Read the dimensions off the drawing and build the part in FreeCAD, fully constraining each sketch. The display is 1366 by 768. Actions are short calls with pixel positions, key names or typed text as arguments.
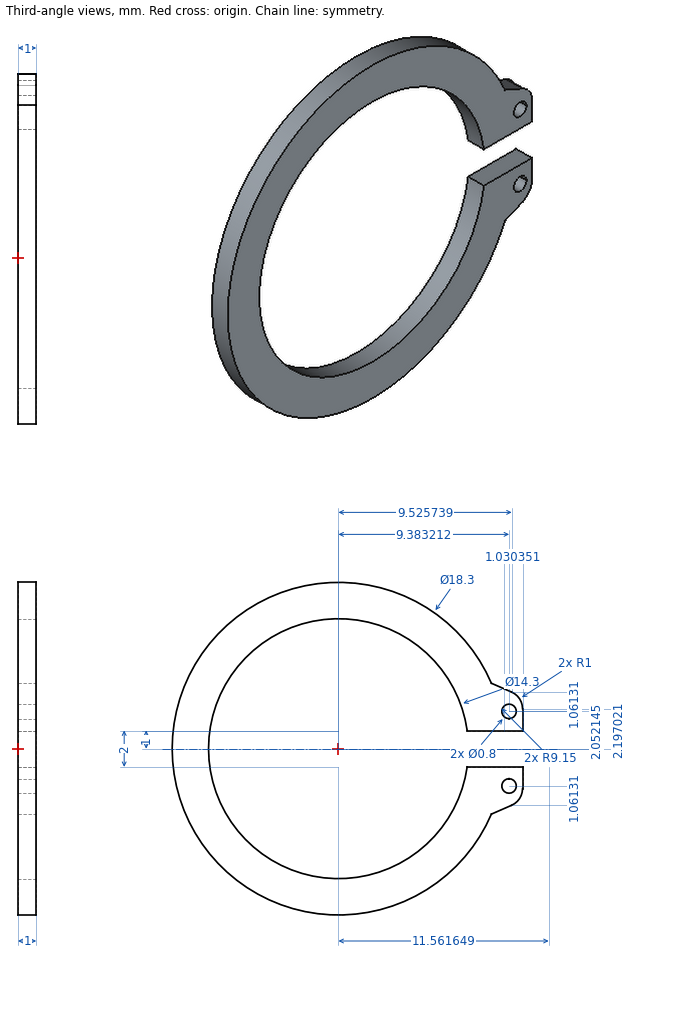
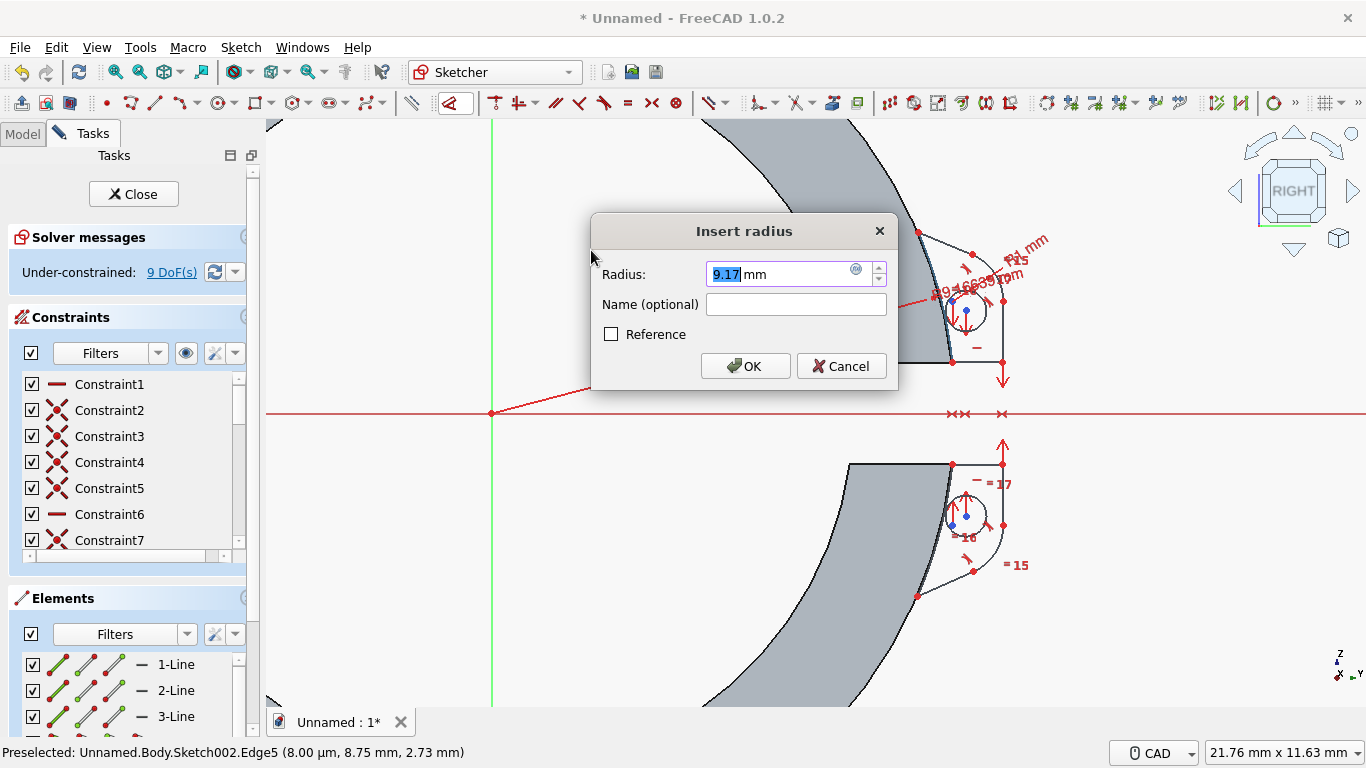
text(9.15)
key(Return)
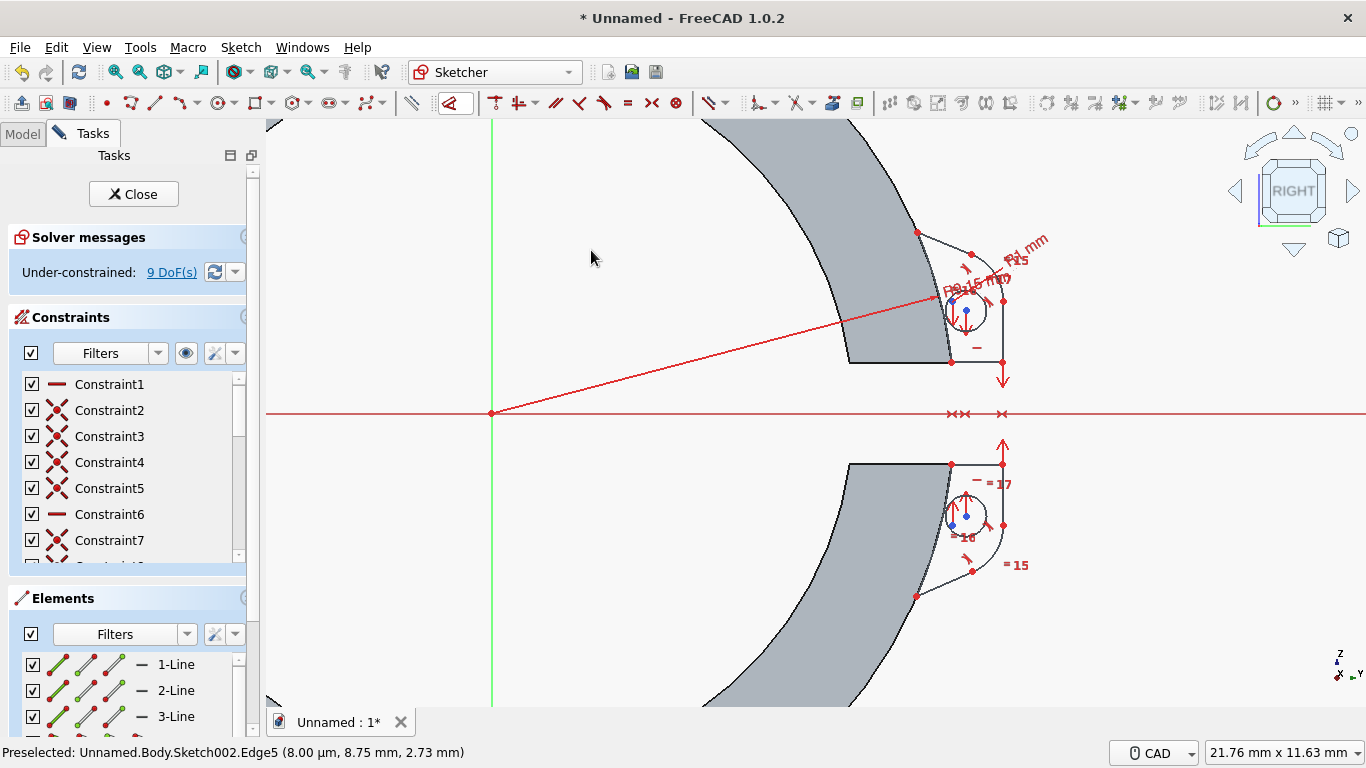
click(980, 296)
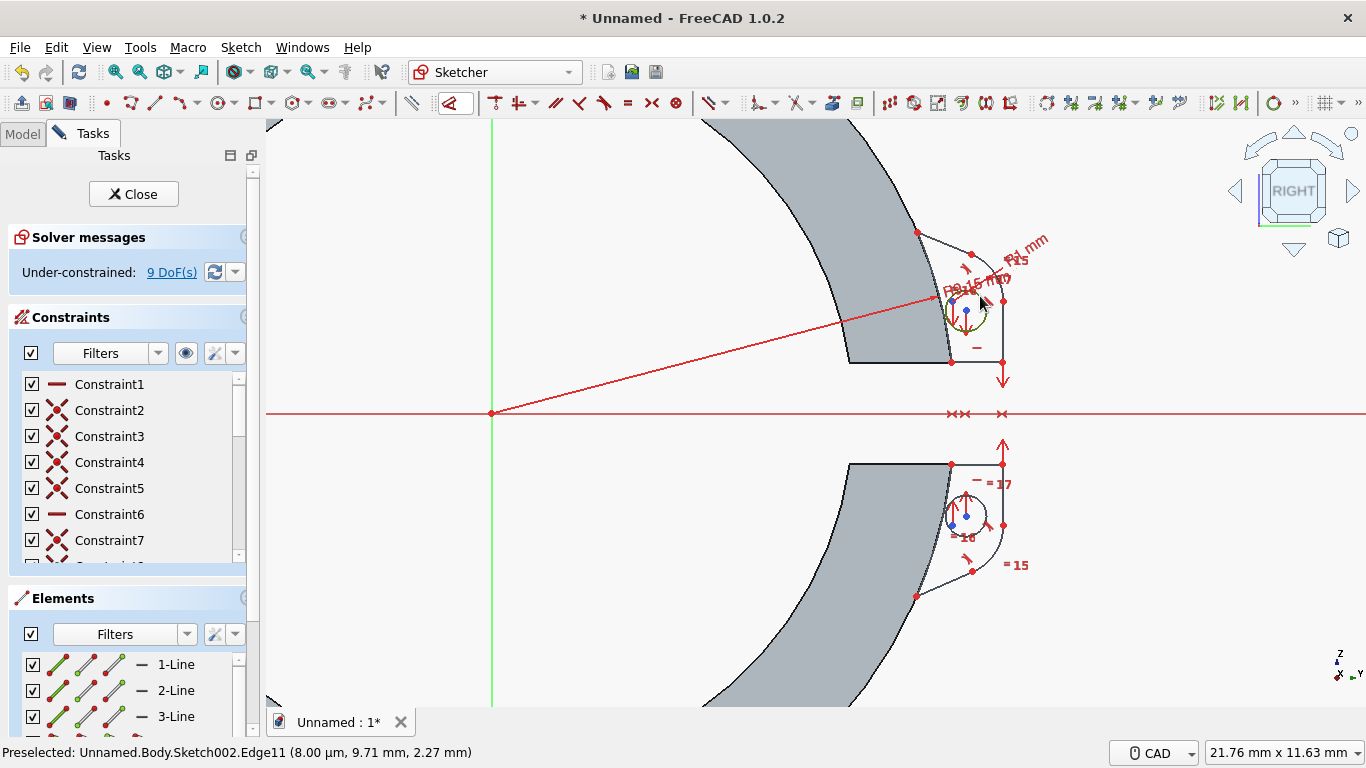
key(k)
key(o)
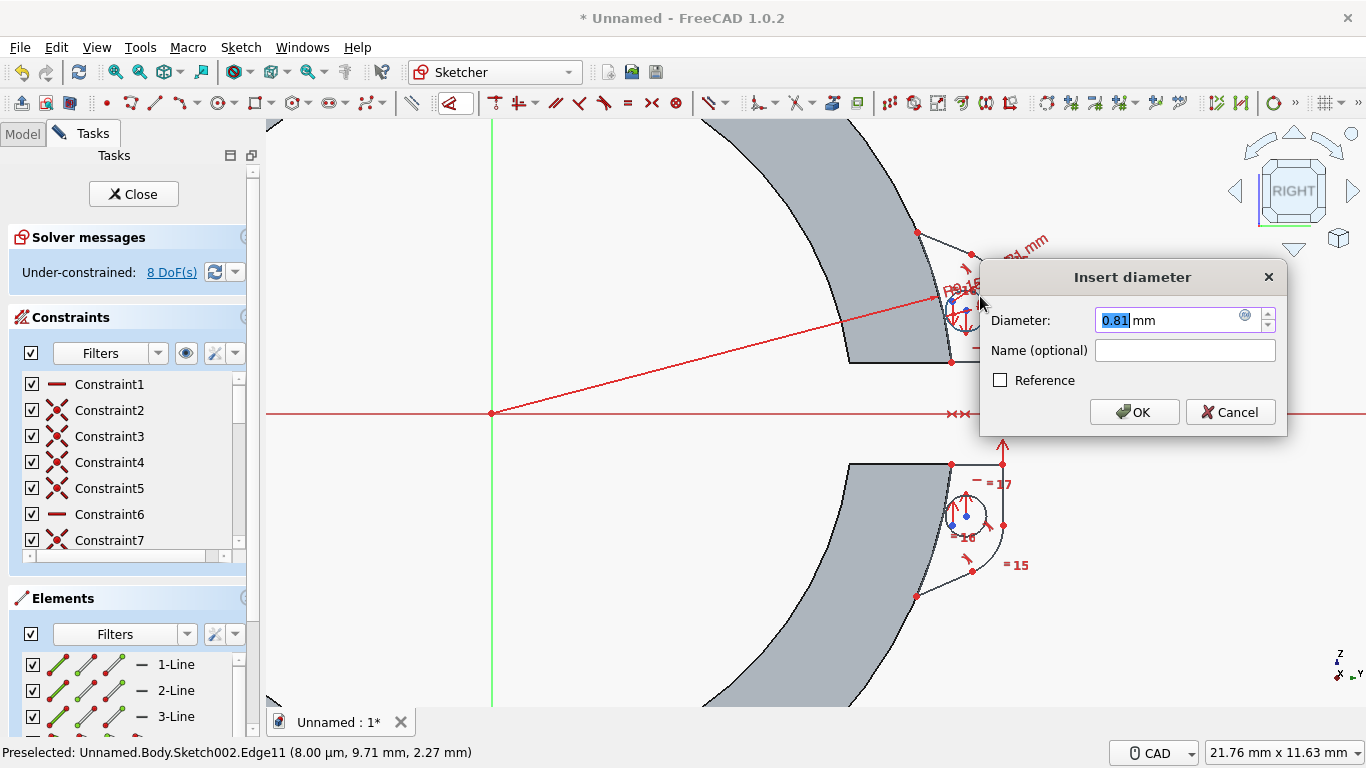
text(0.8)
key(Return)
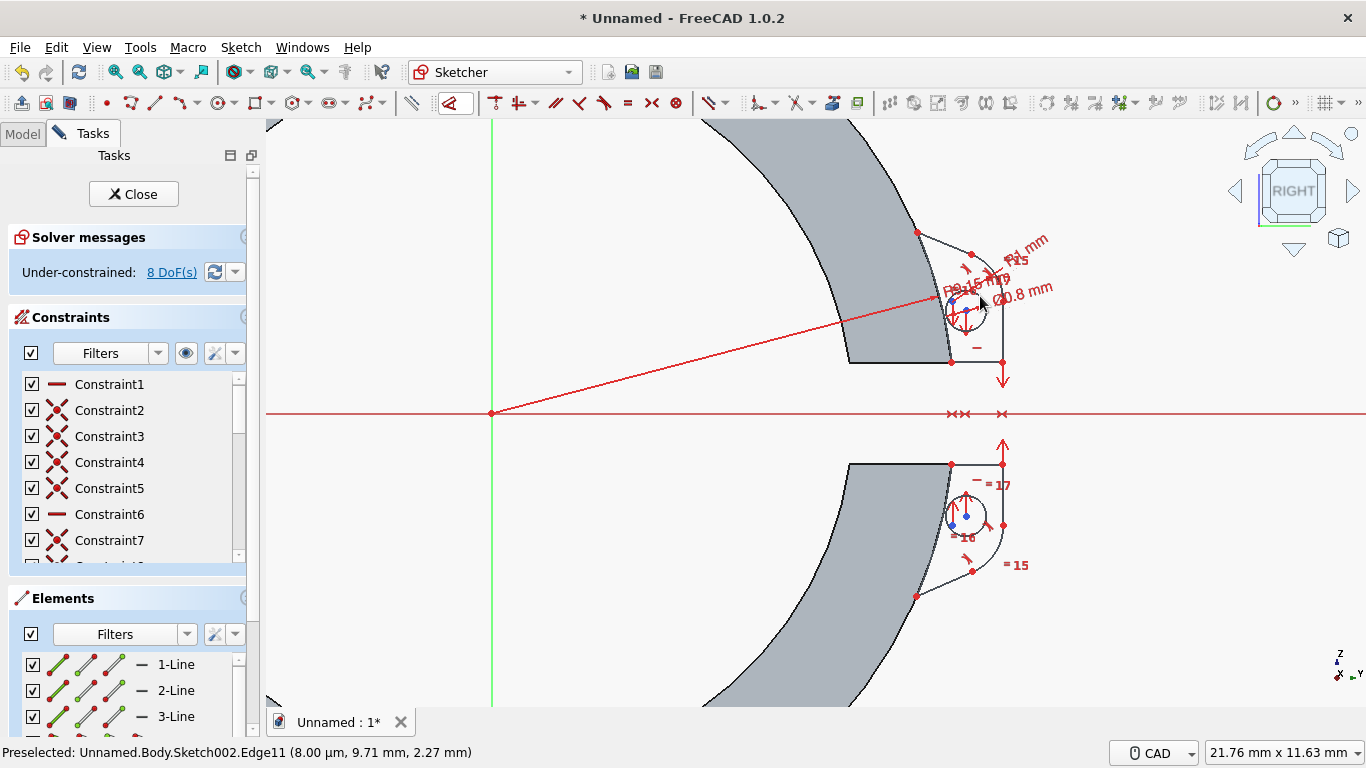
click(952, 362)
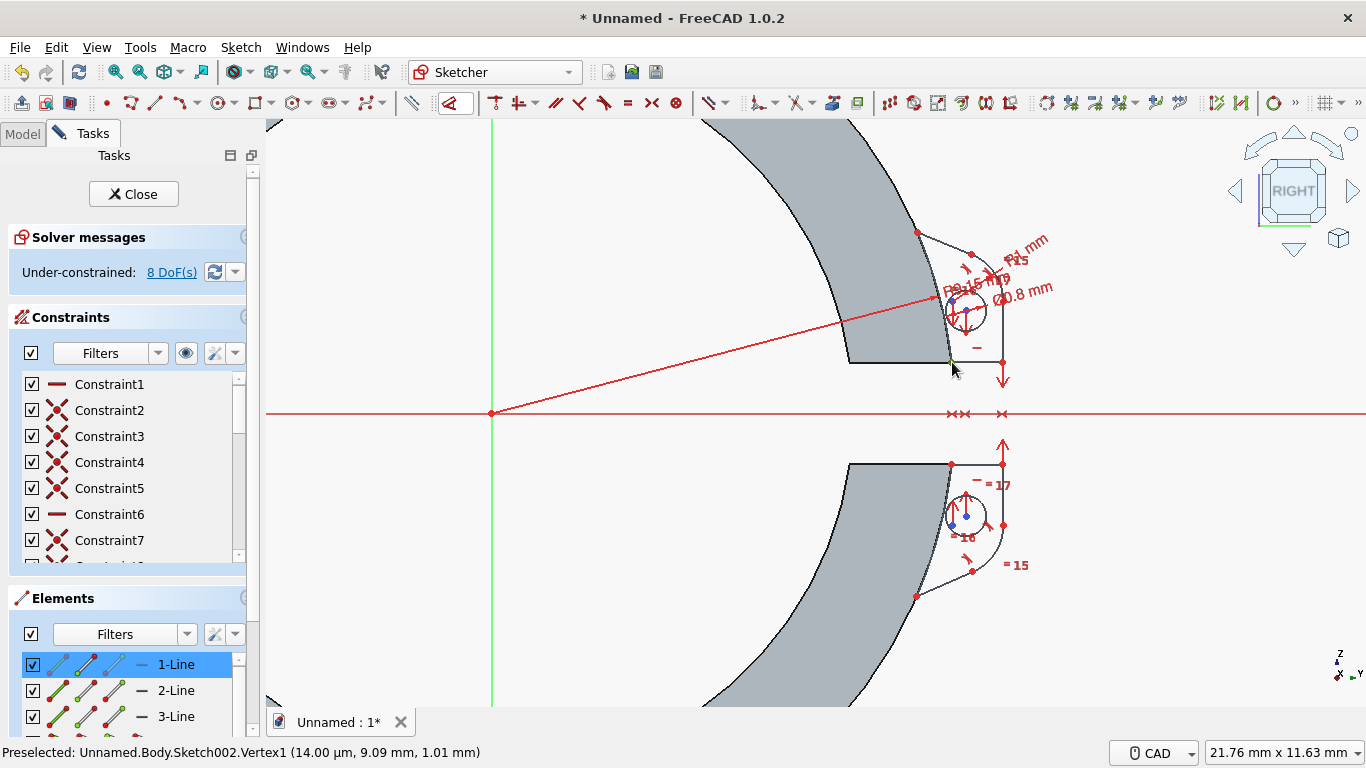
key(i)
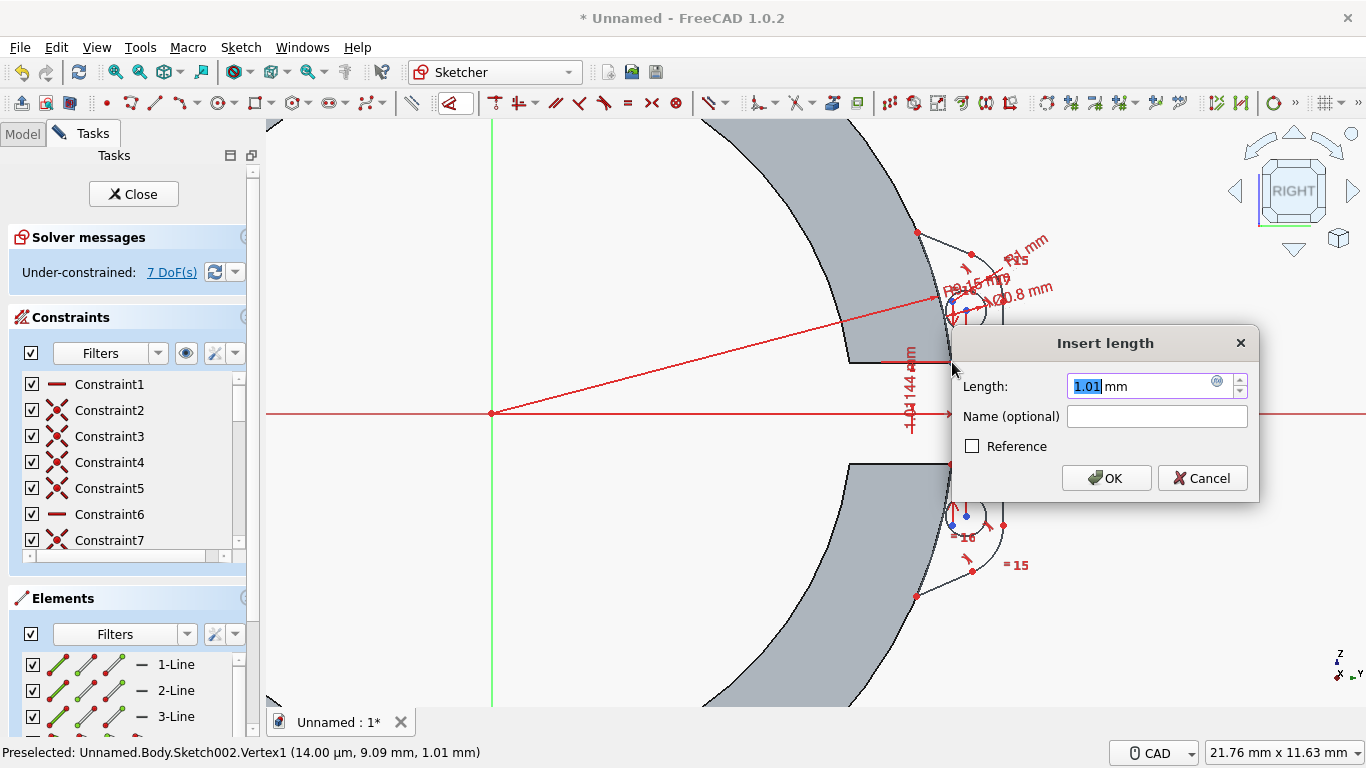
text(1)
key(Return)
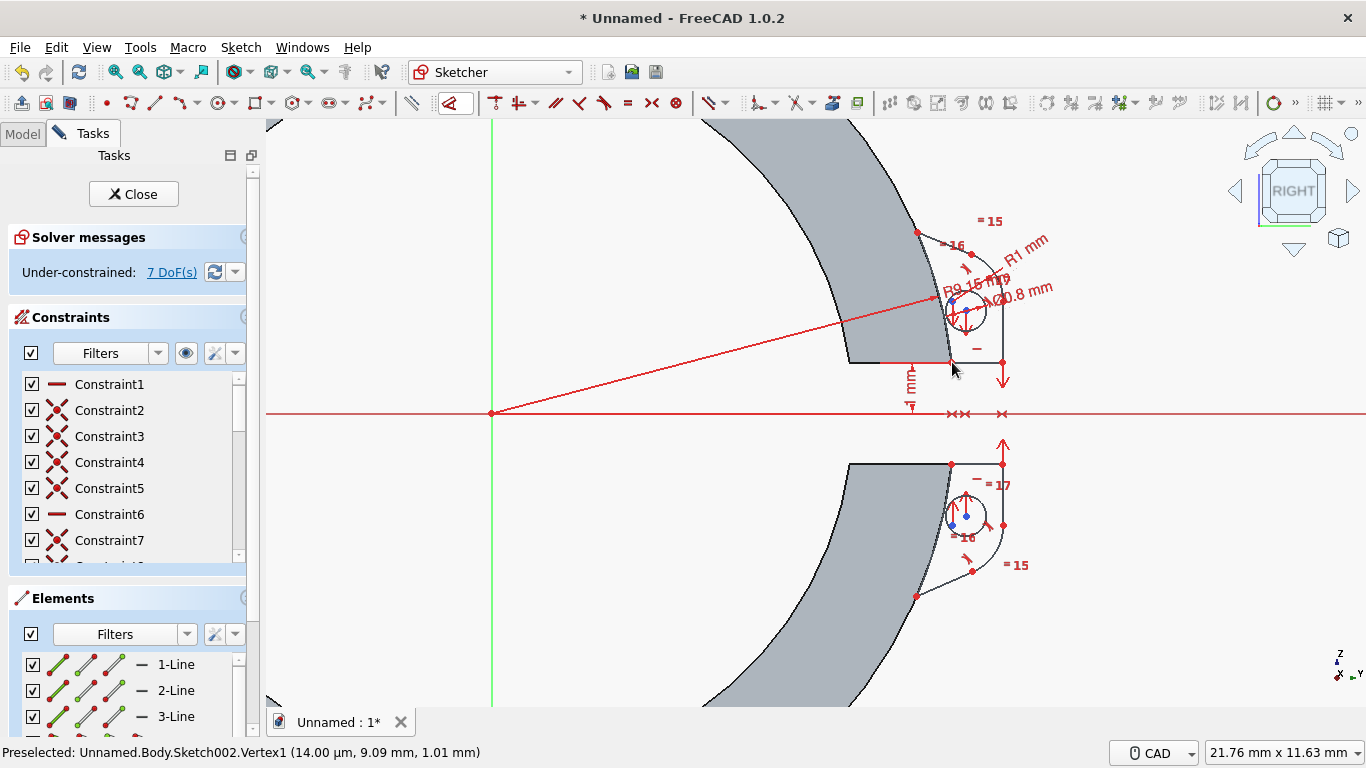
click(967, 363)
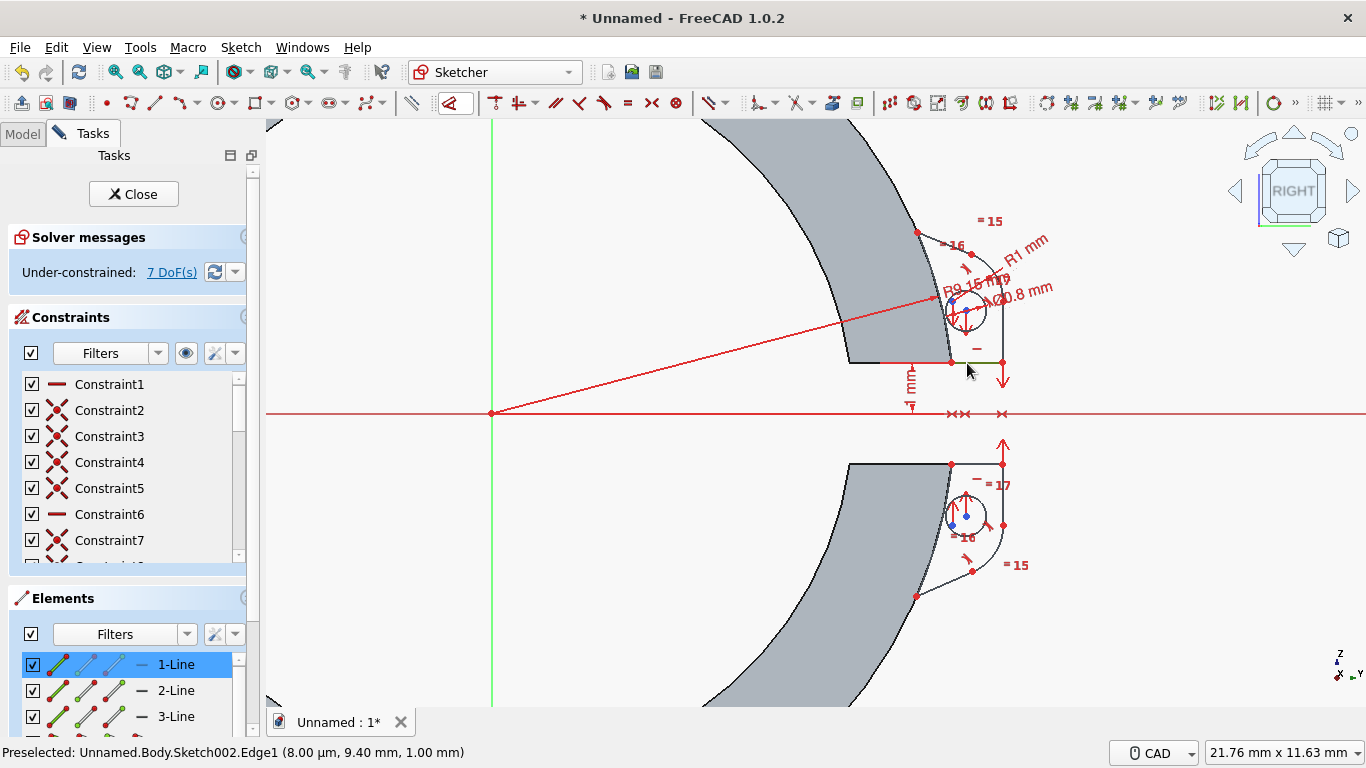
key(l)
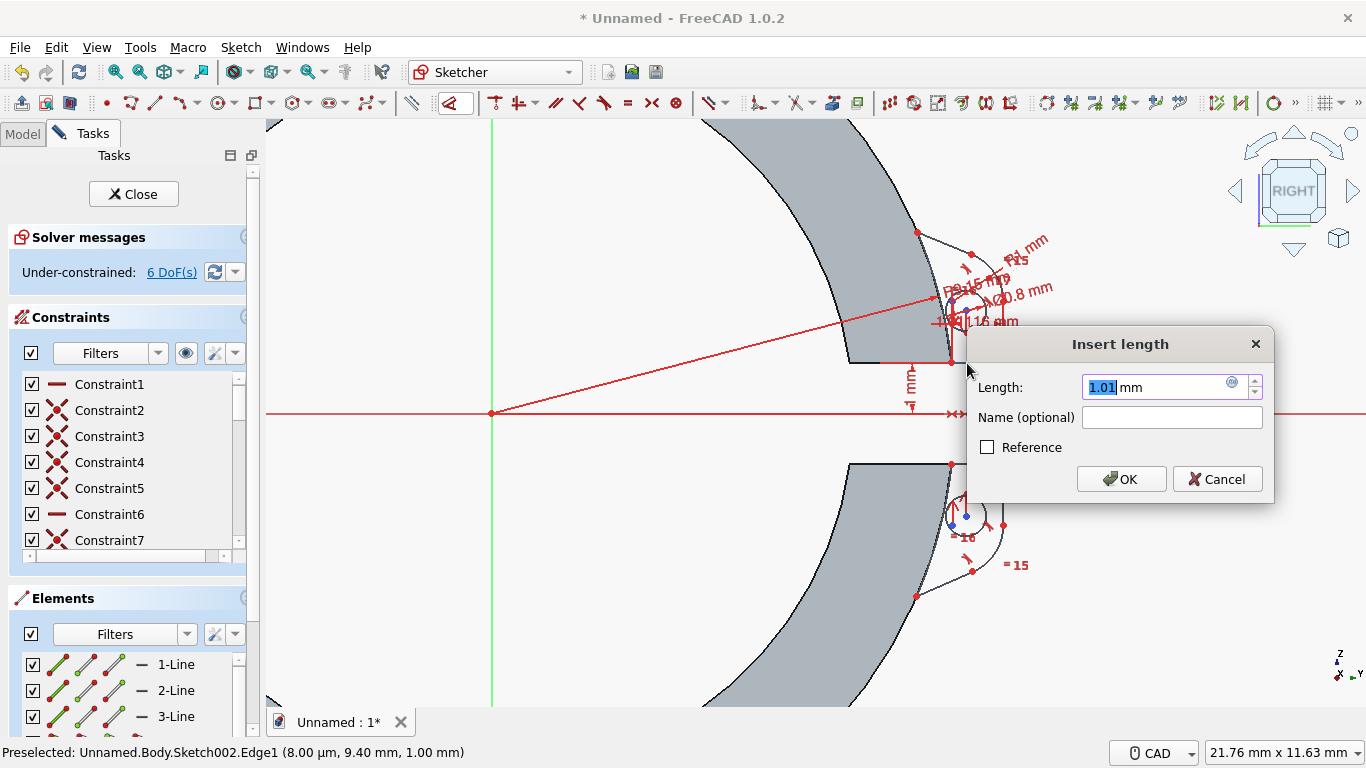
text(1.030351)
key(Return)